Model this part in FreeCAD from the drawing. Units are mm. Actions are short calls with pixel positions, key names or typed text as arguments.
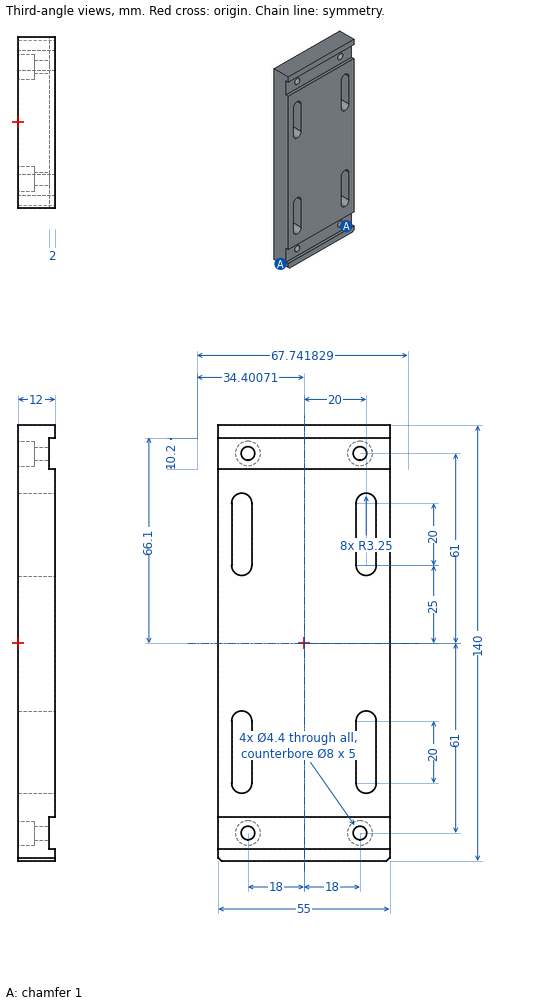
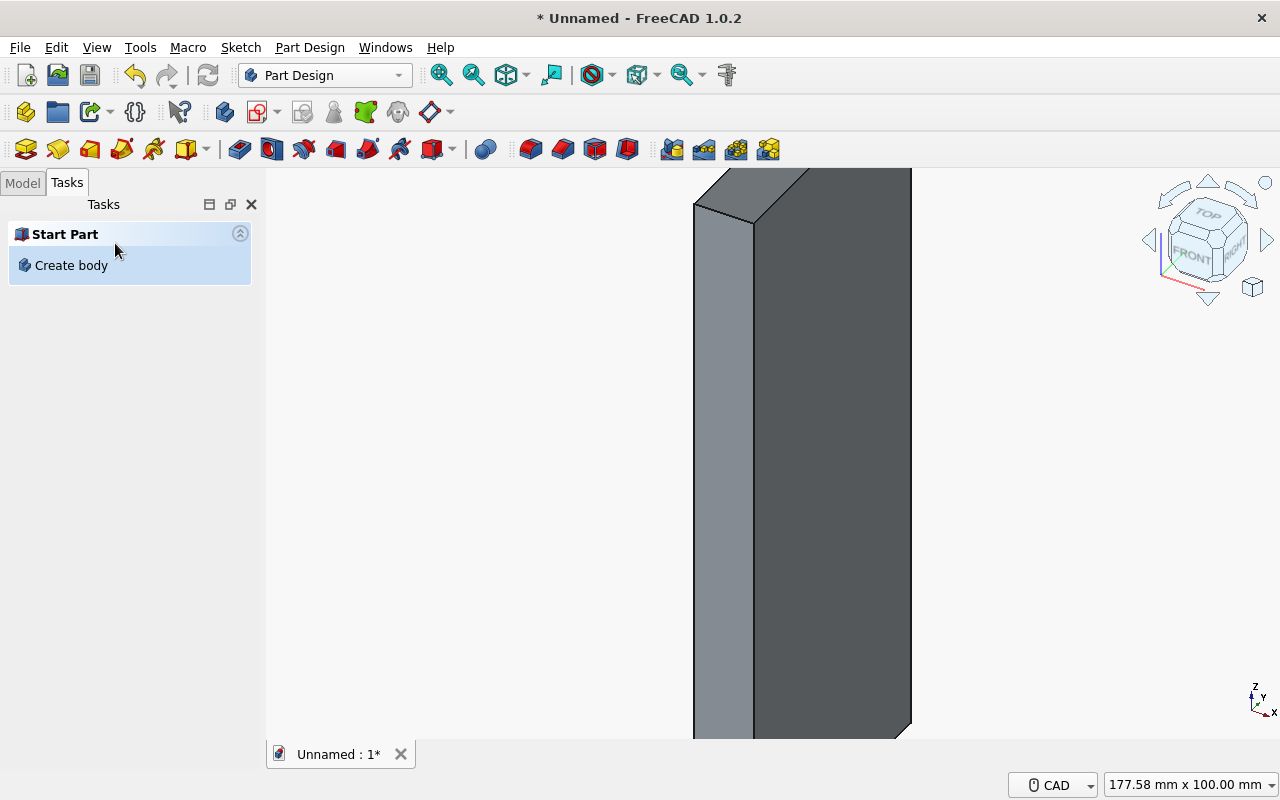
click(442, 76)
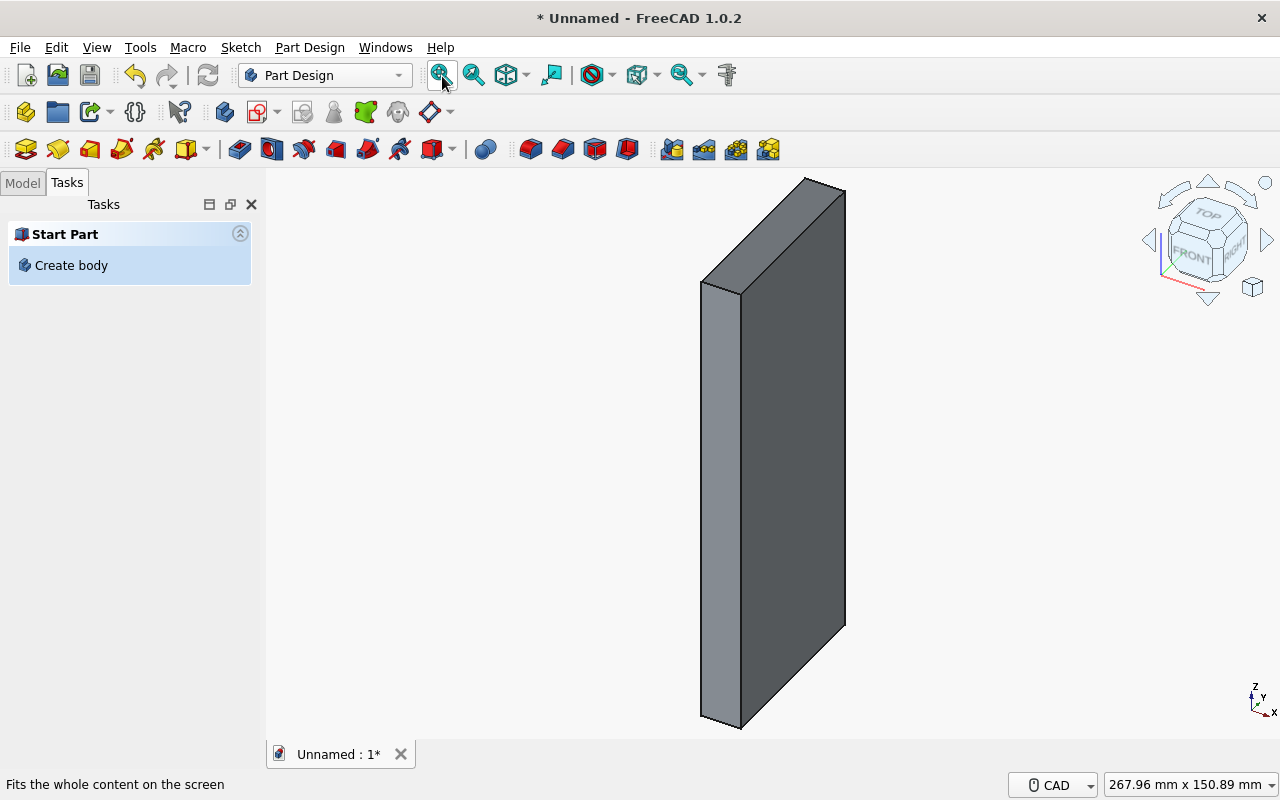
click(793, 583)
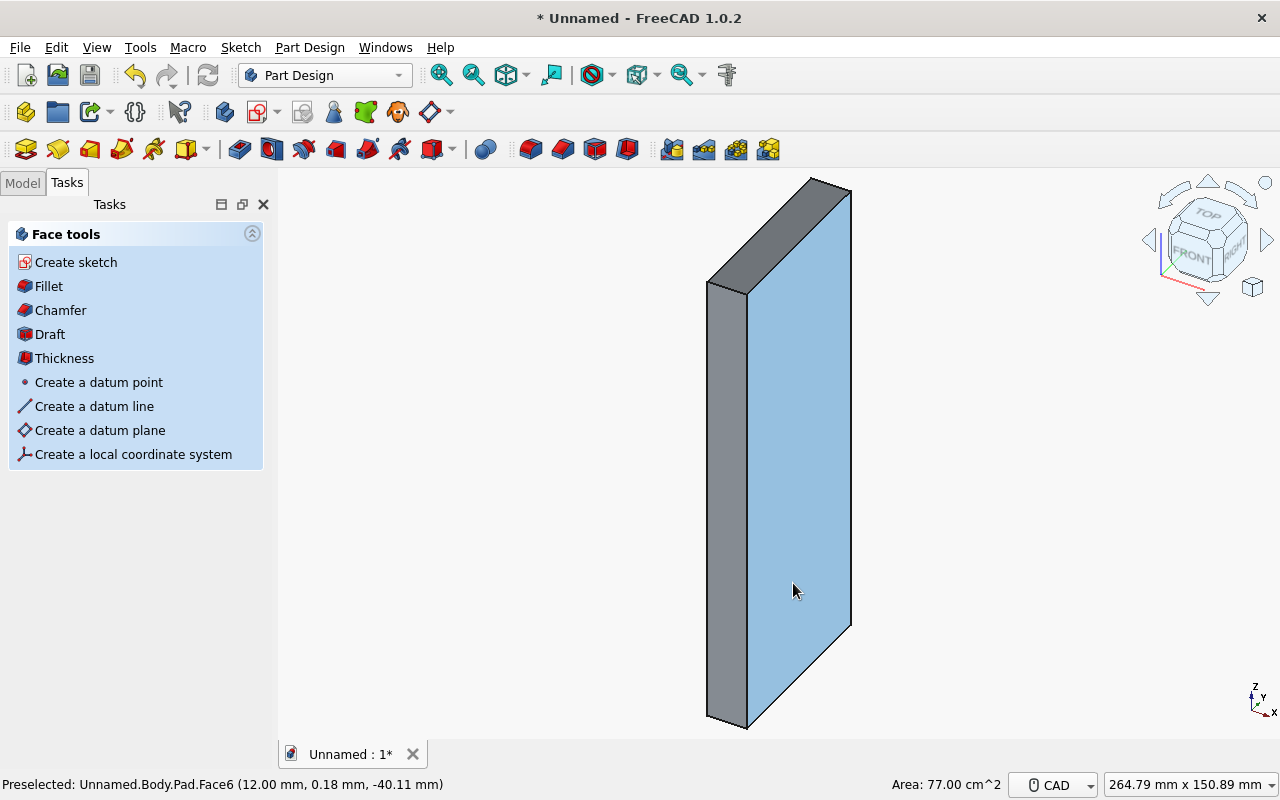
click(258, 112)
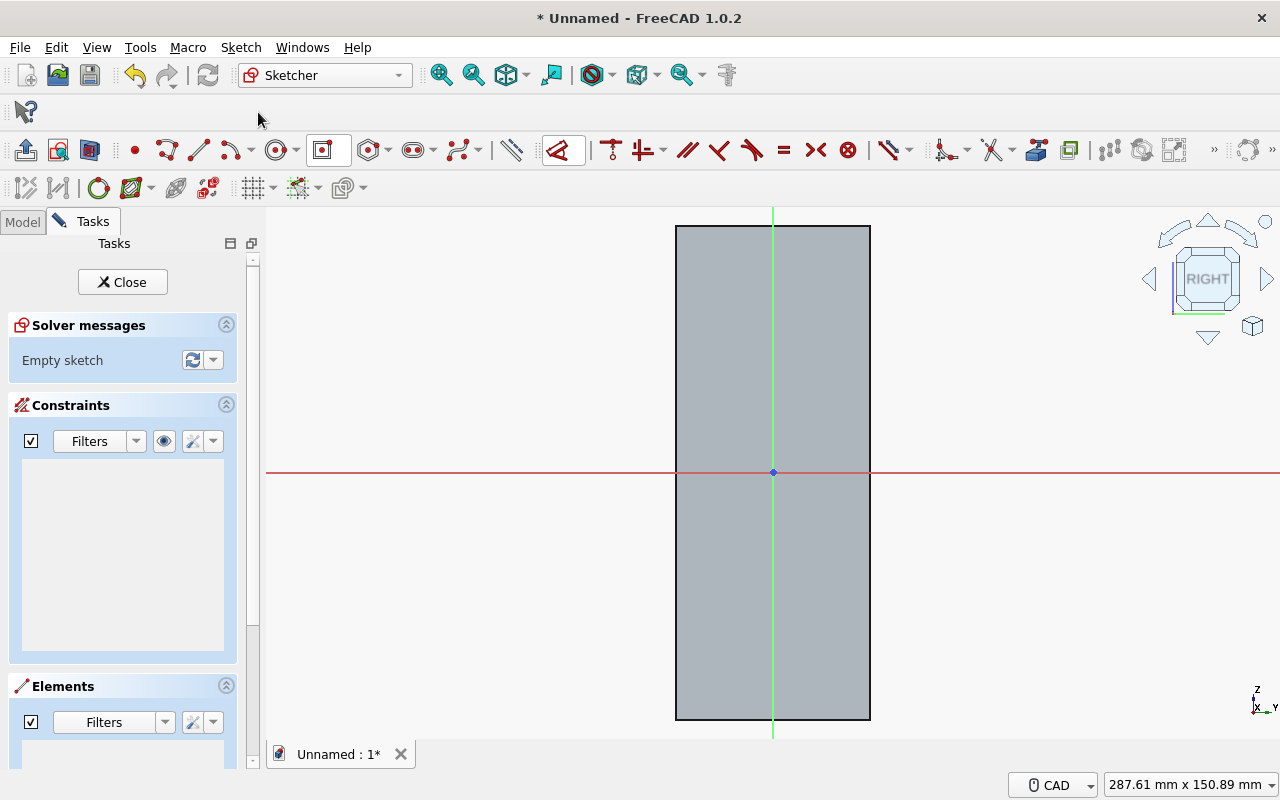
scroll(404, 711, down, 1)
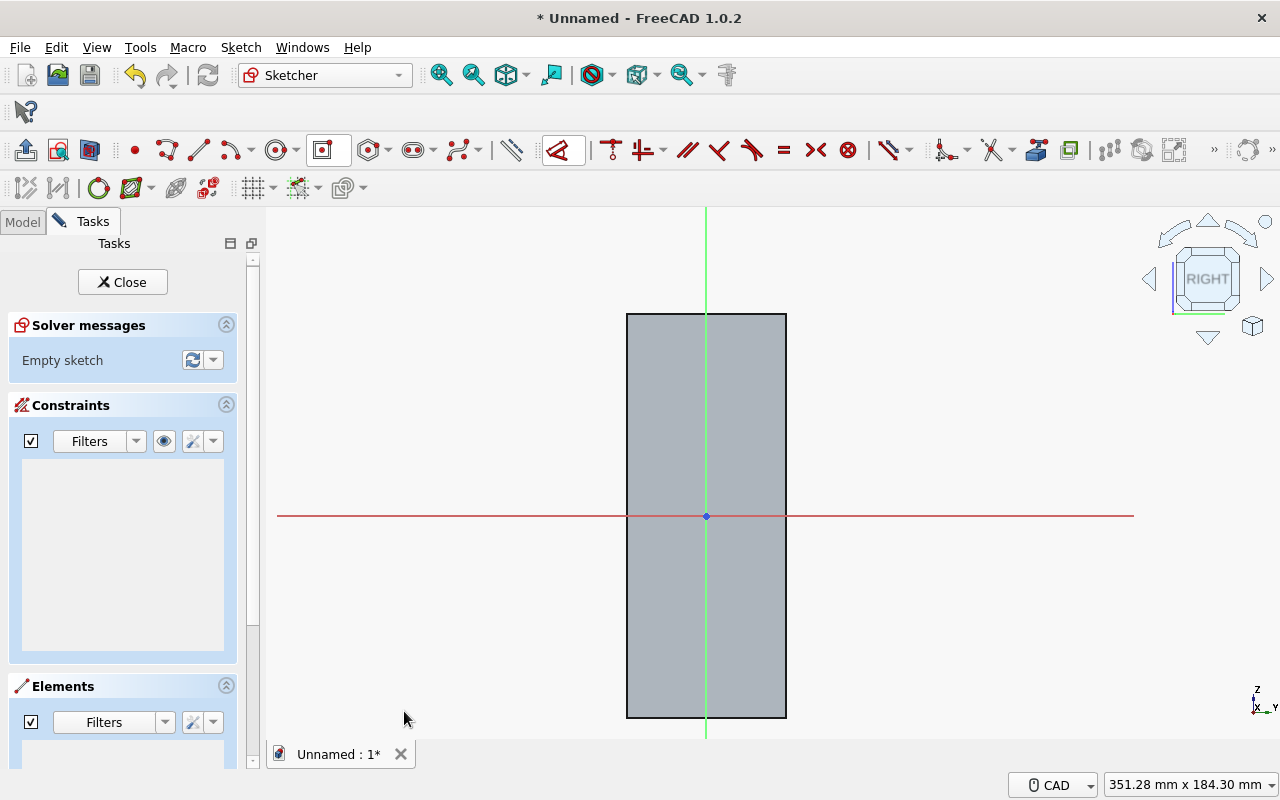
scroll(705, 358, up, 3)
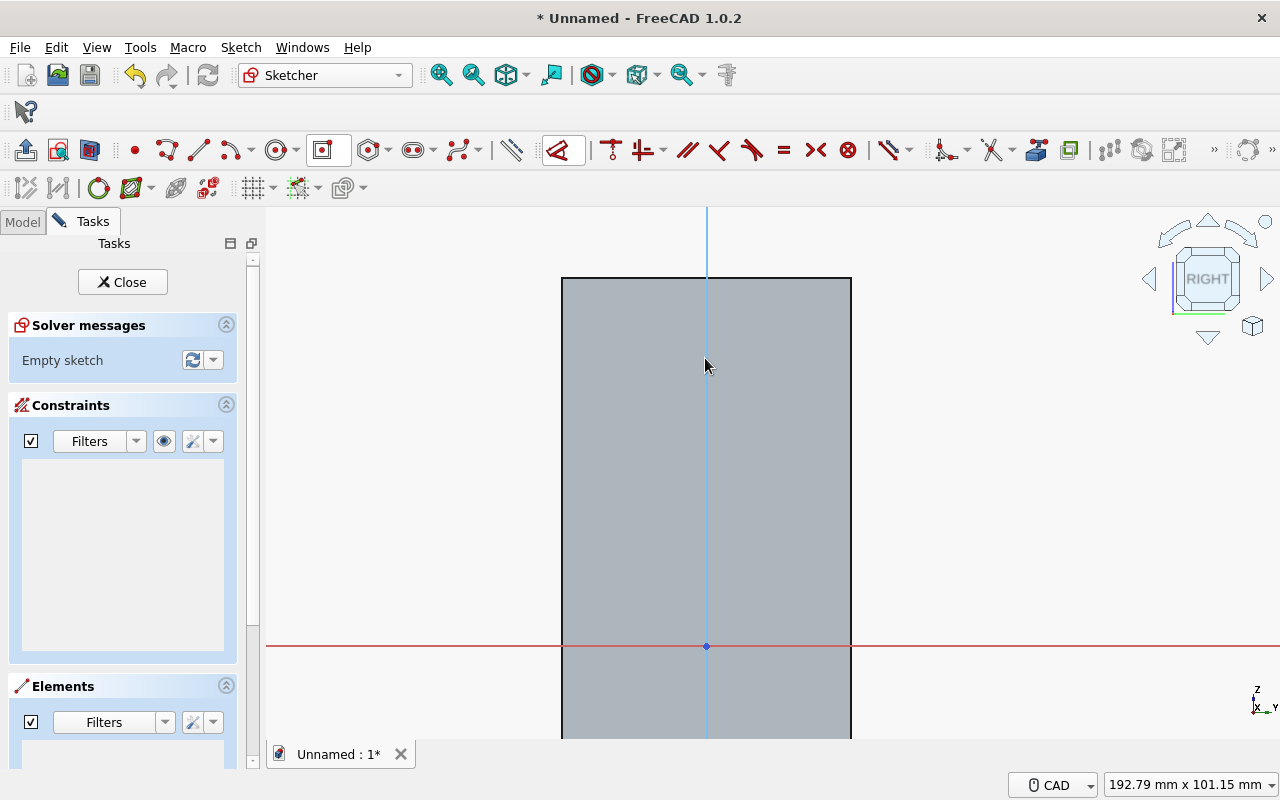
click(346, 150)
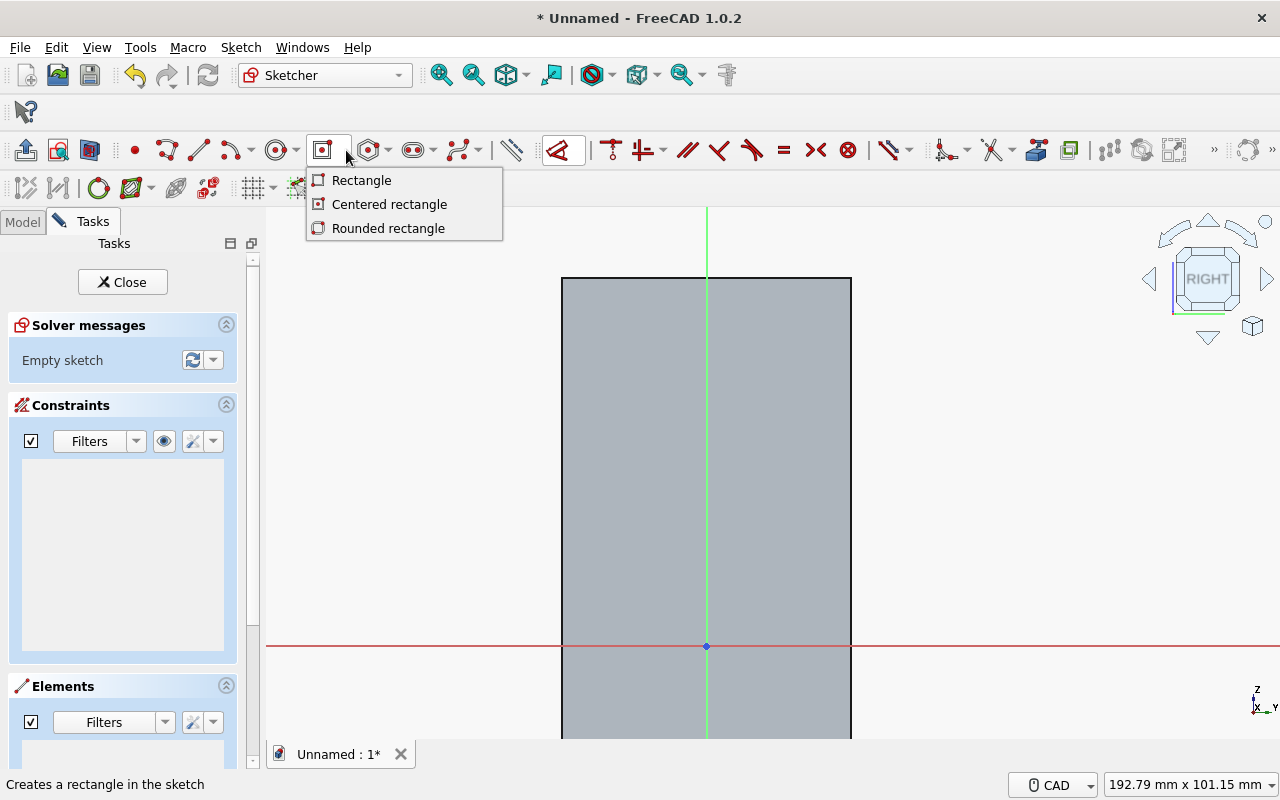
click(404, 180)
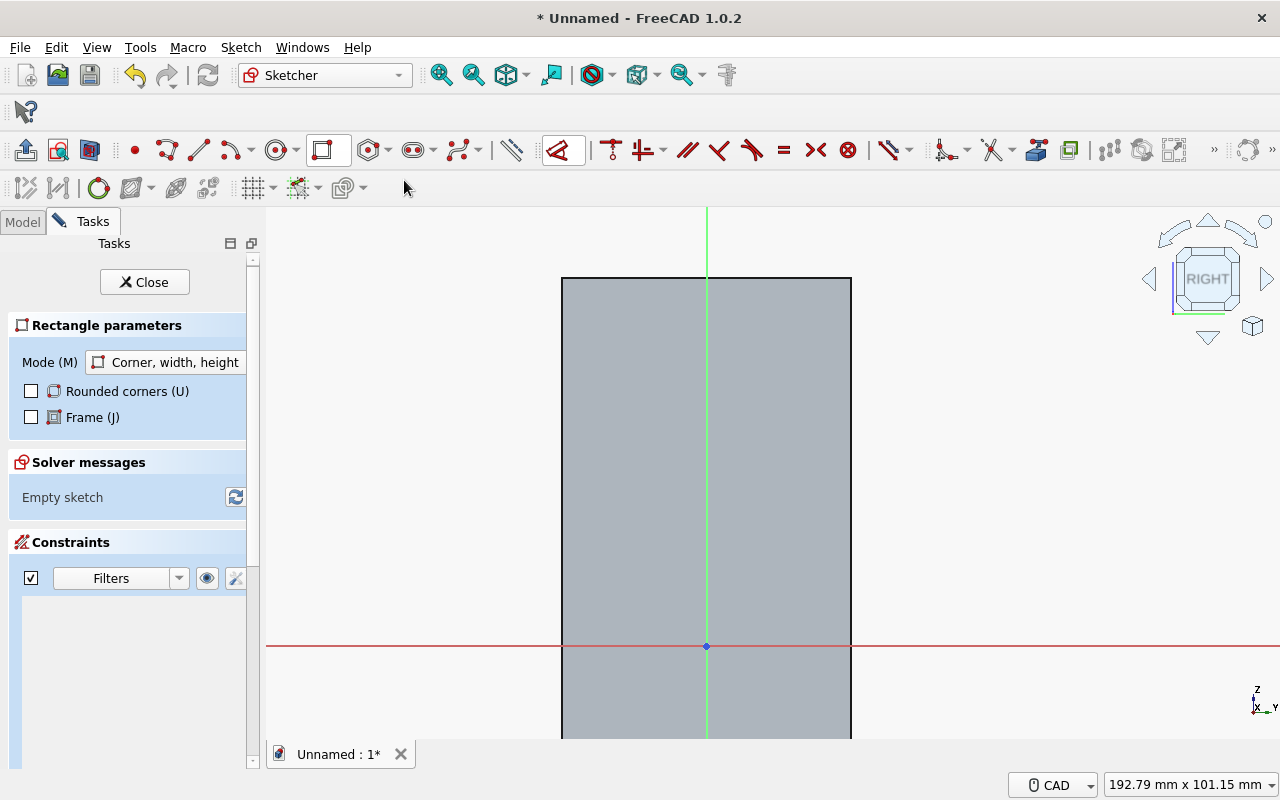
click(526, 299)
click(882, 352)
key(Escape)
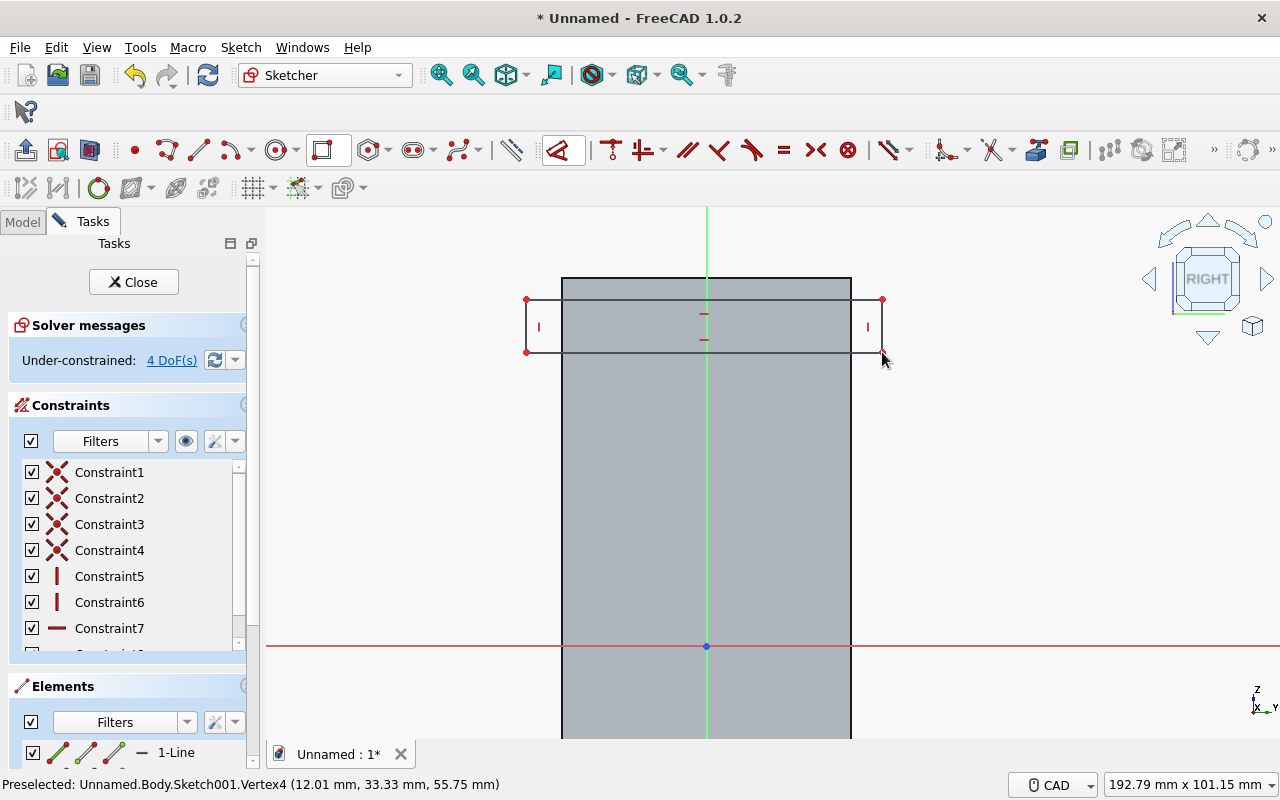
click(526, 316)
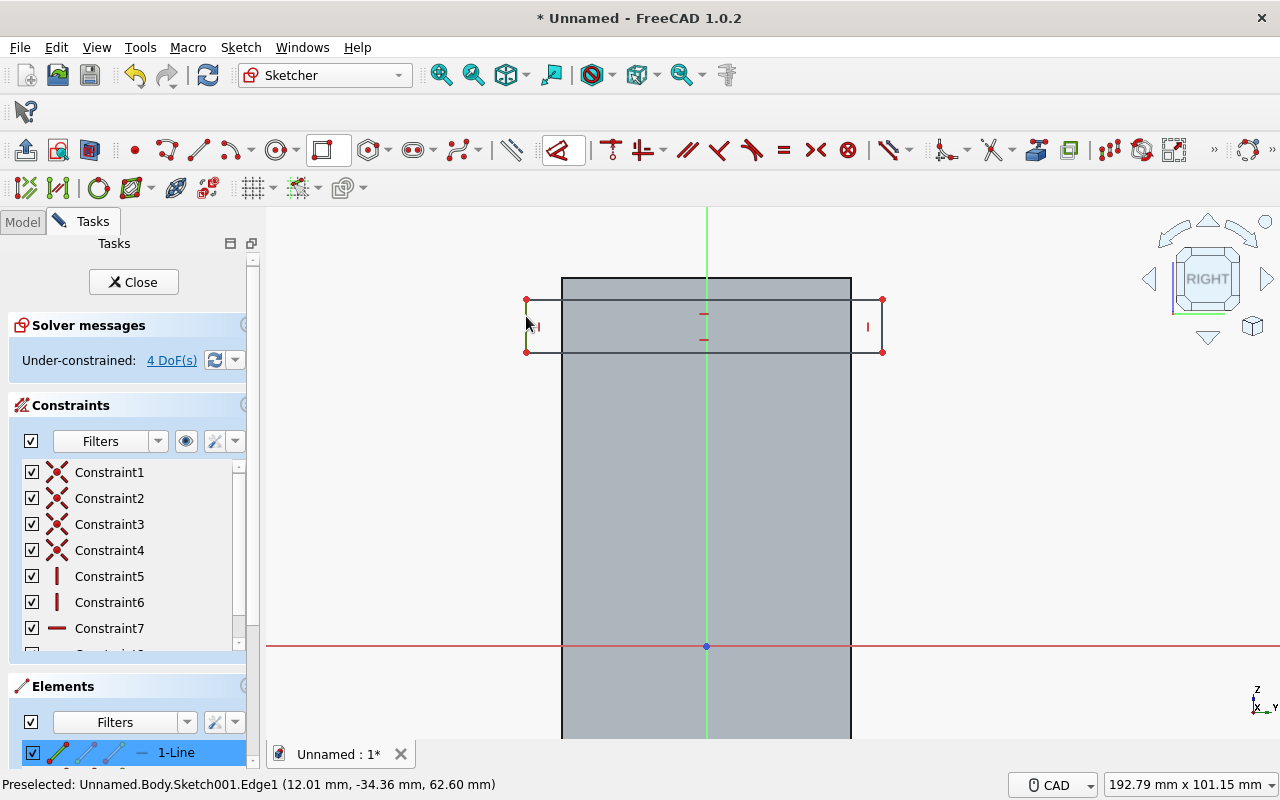
click(580, 150)